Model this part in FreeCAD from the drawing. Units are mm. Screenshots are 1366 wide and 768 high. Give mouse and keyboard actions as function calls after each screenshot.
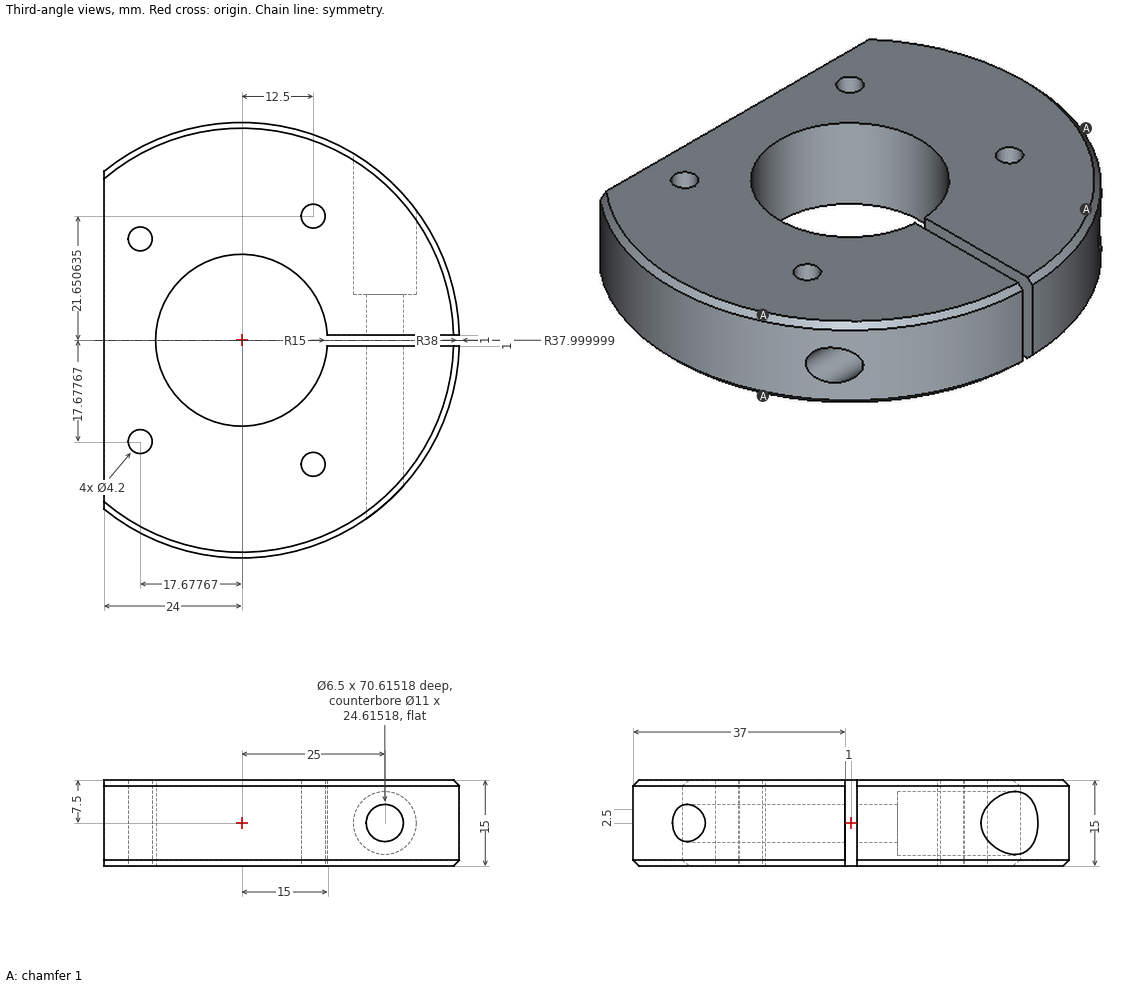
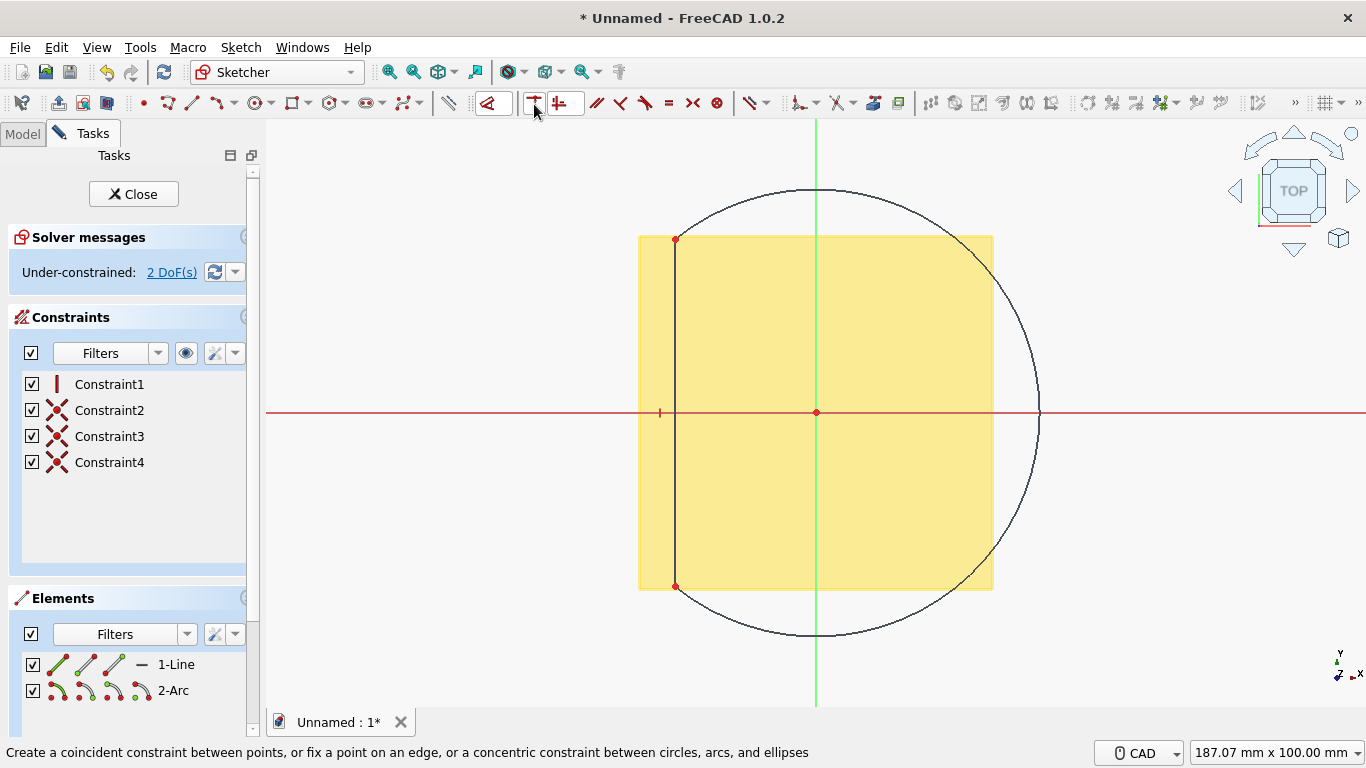
click(488, 104)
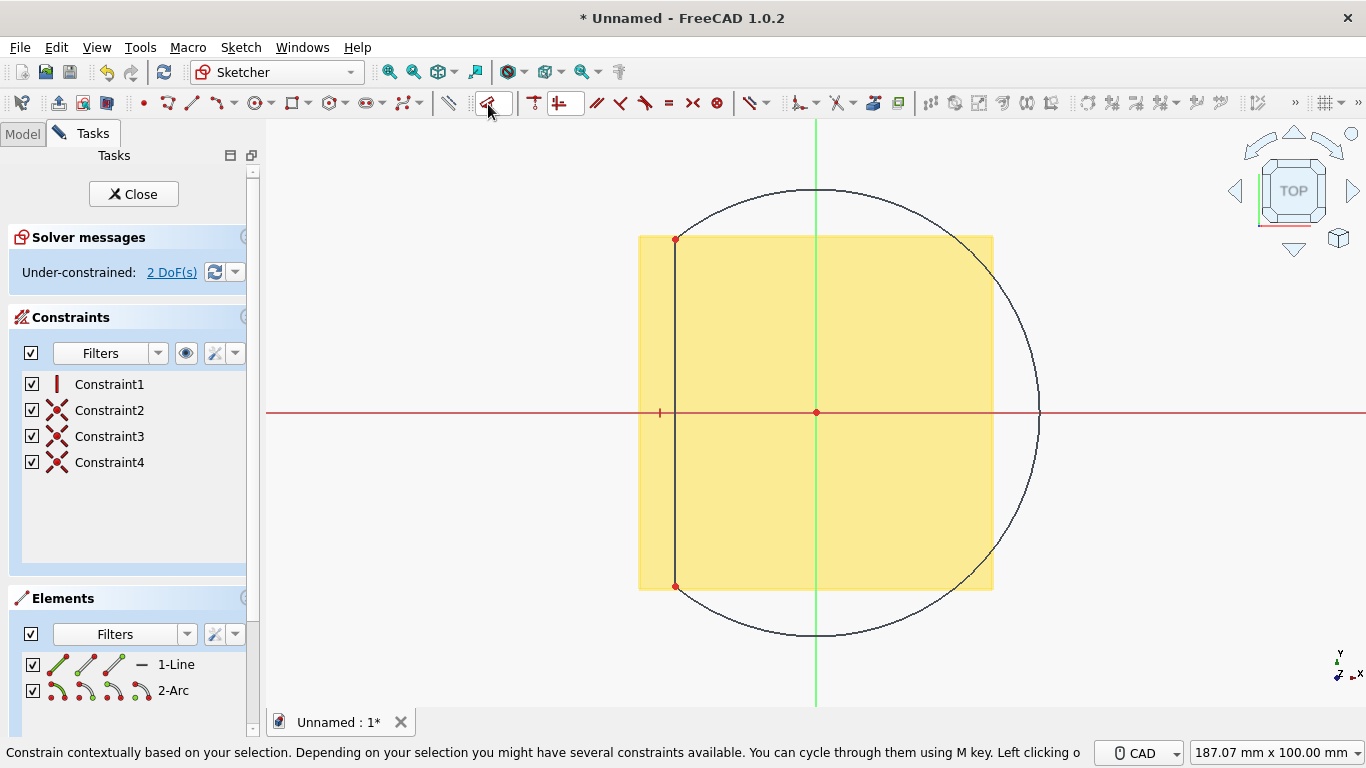
click(955, 588)
click(975, 613)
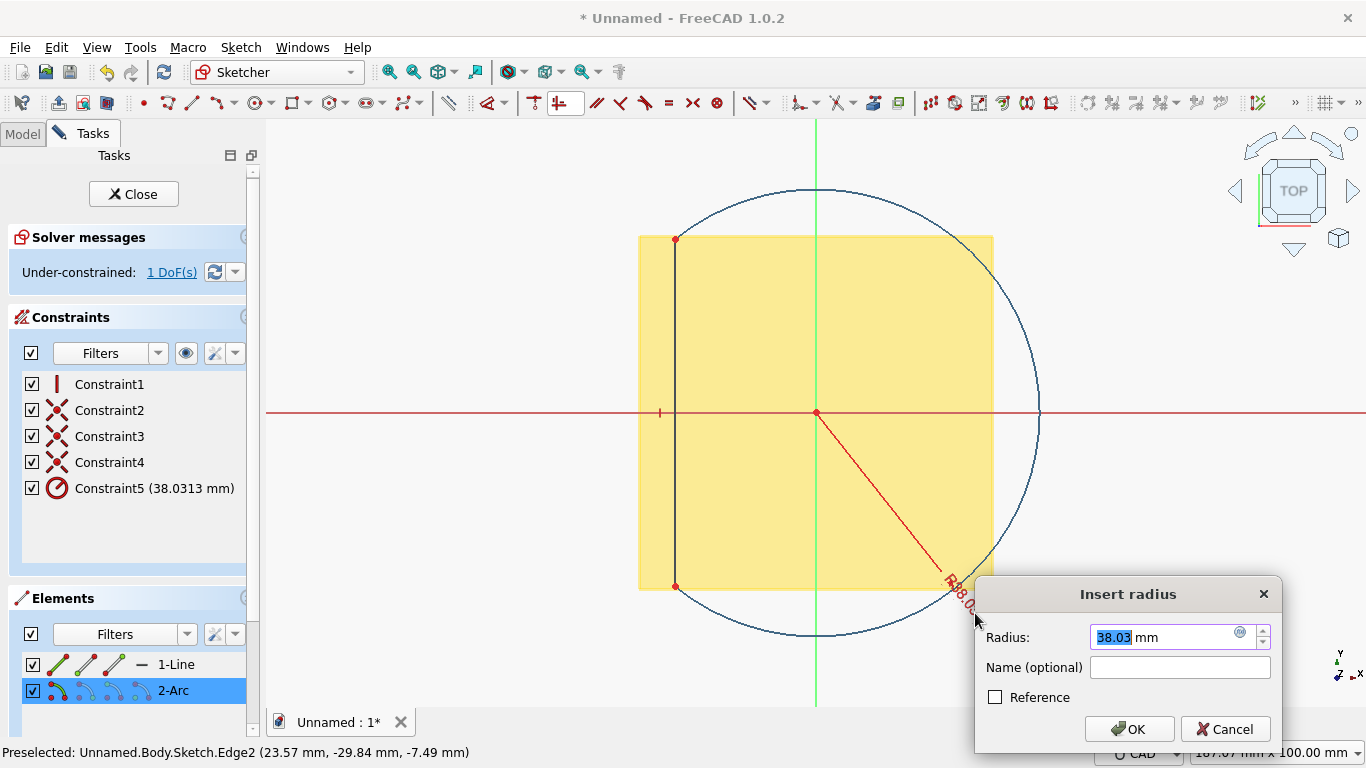
text(38)
key(Return)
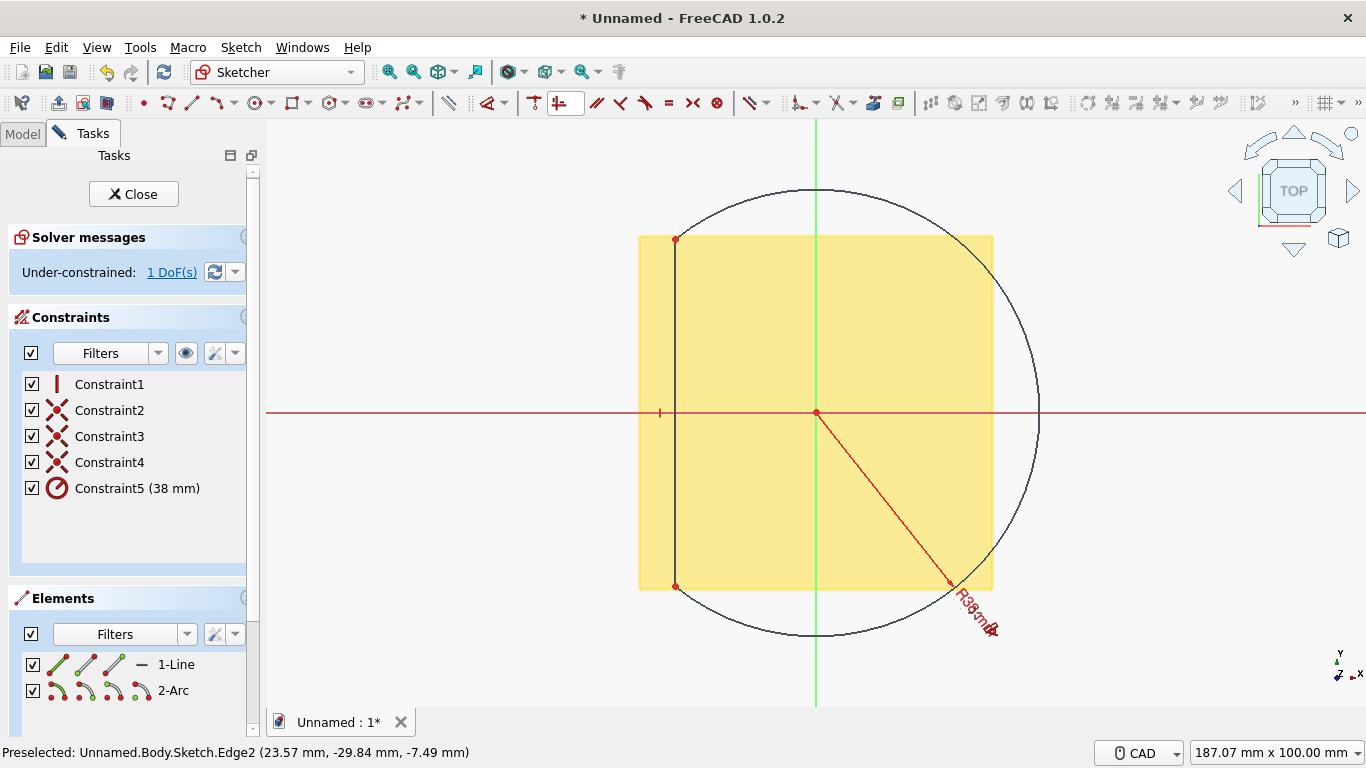
click(675, 587)
click(696, 621)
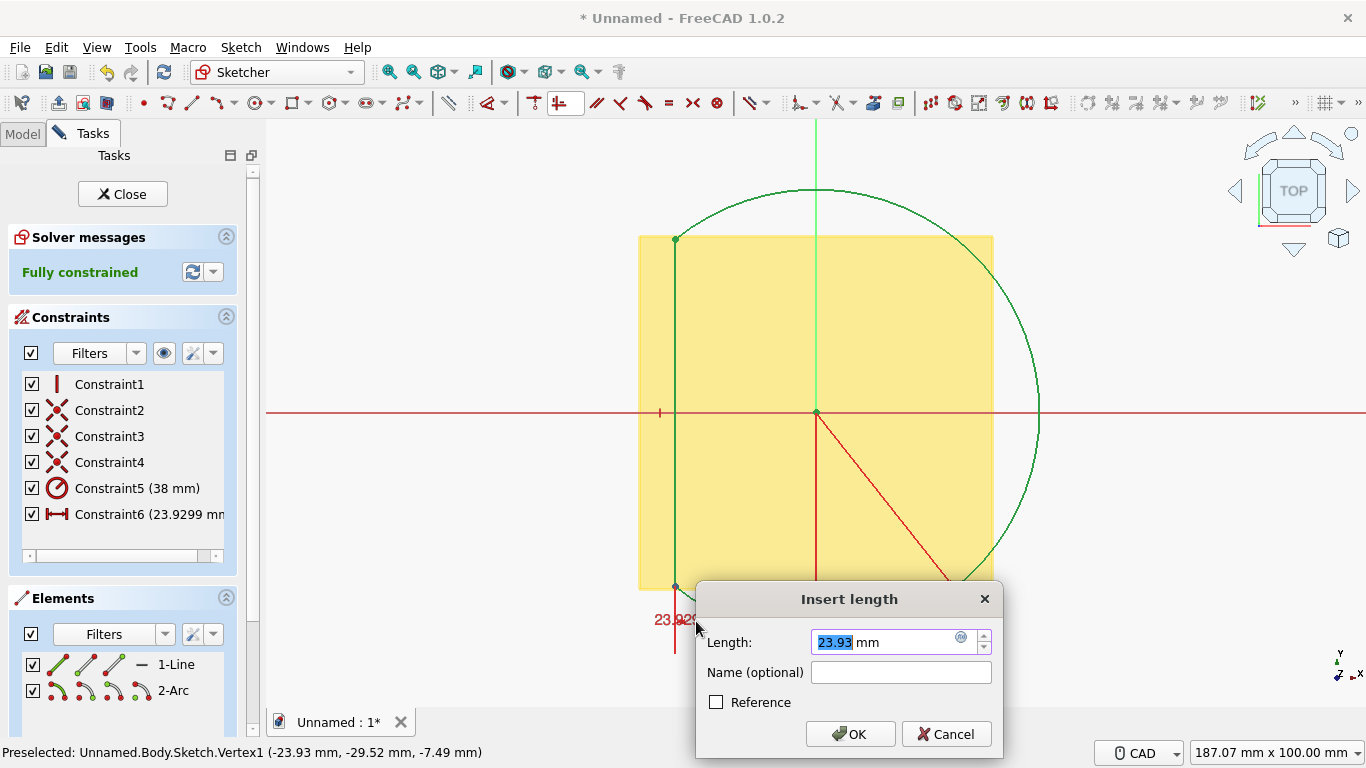
text(24)
key(Return)
key(Escape)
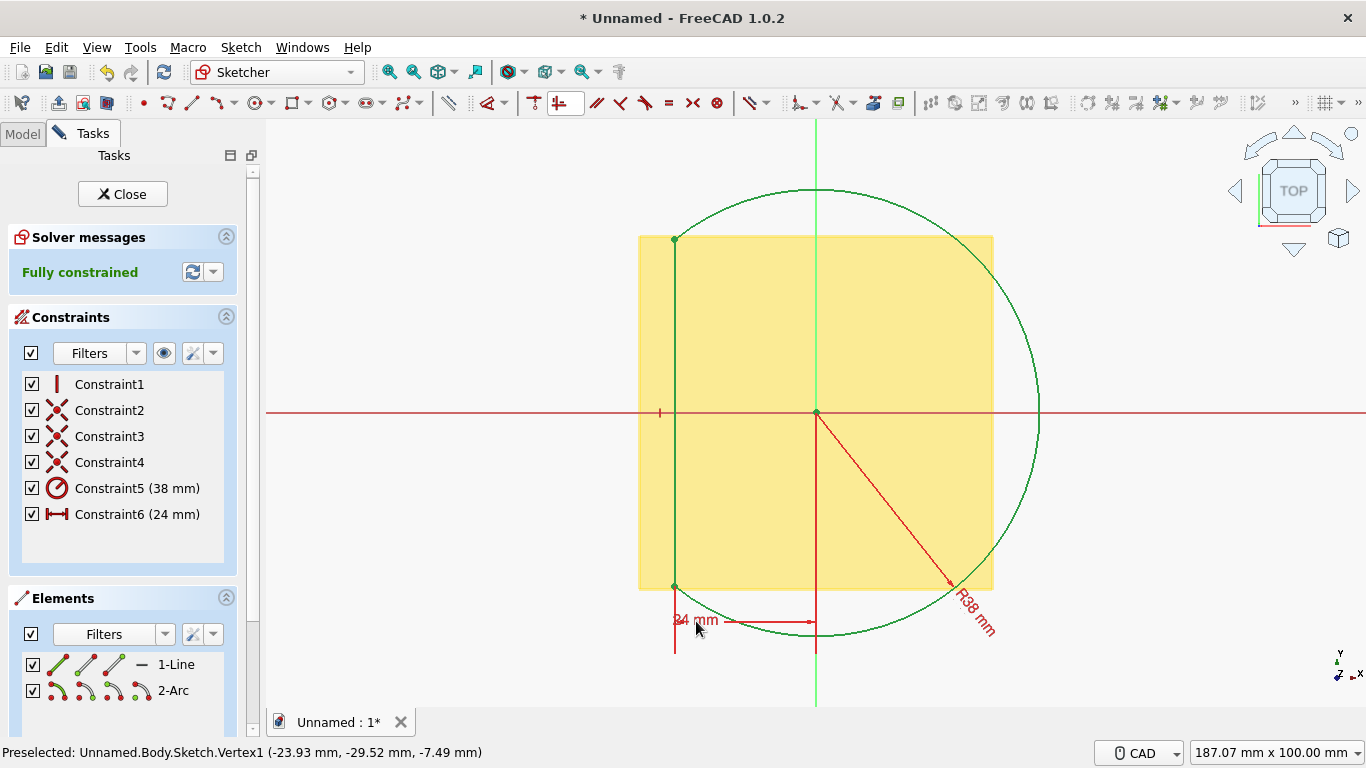
click(123, 194)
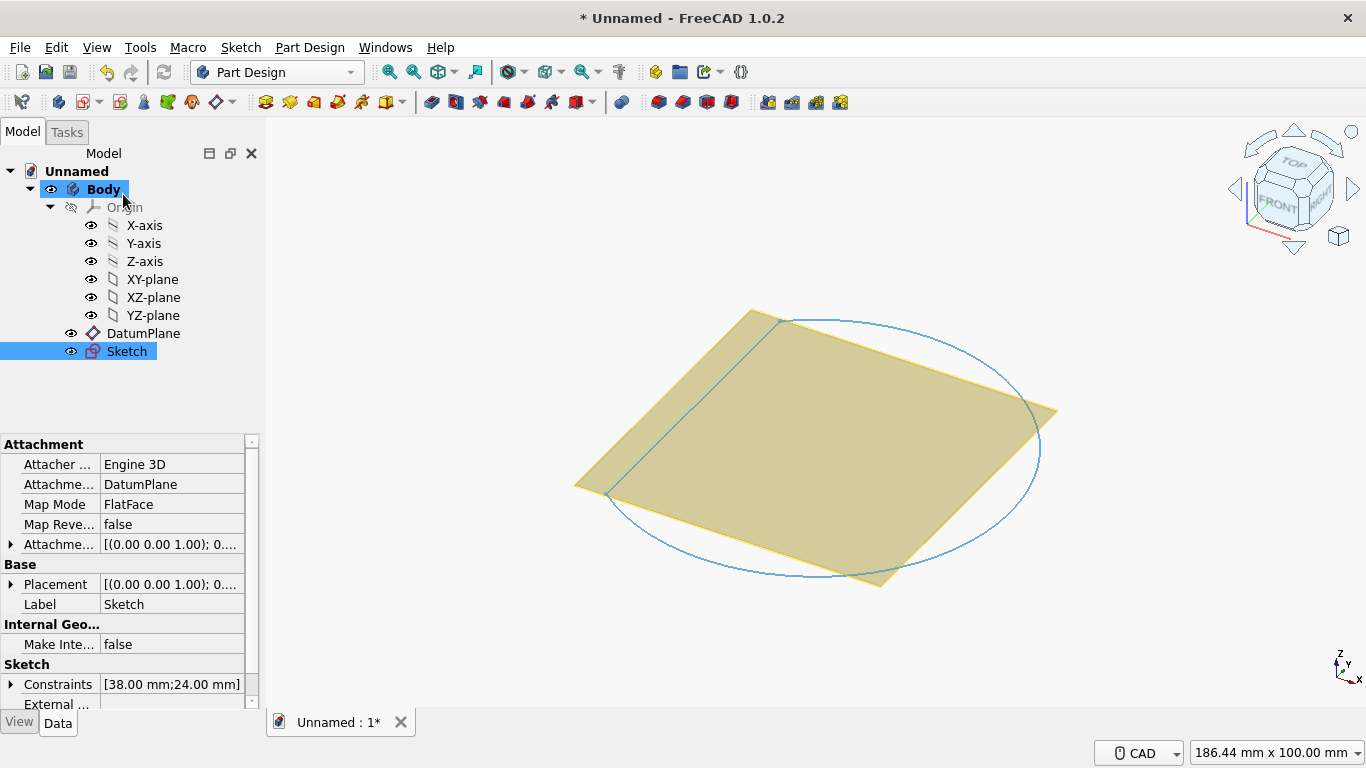
click(266, 102)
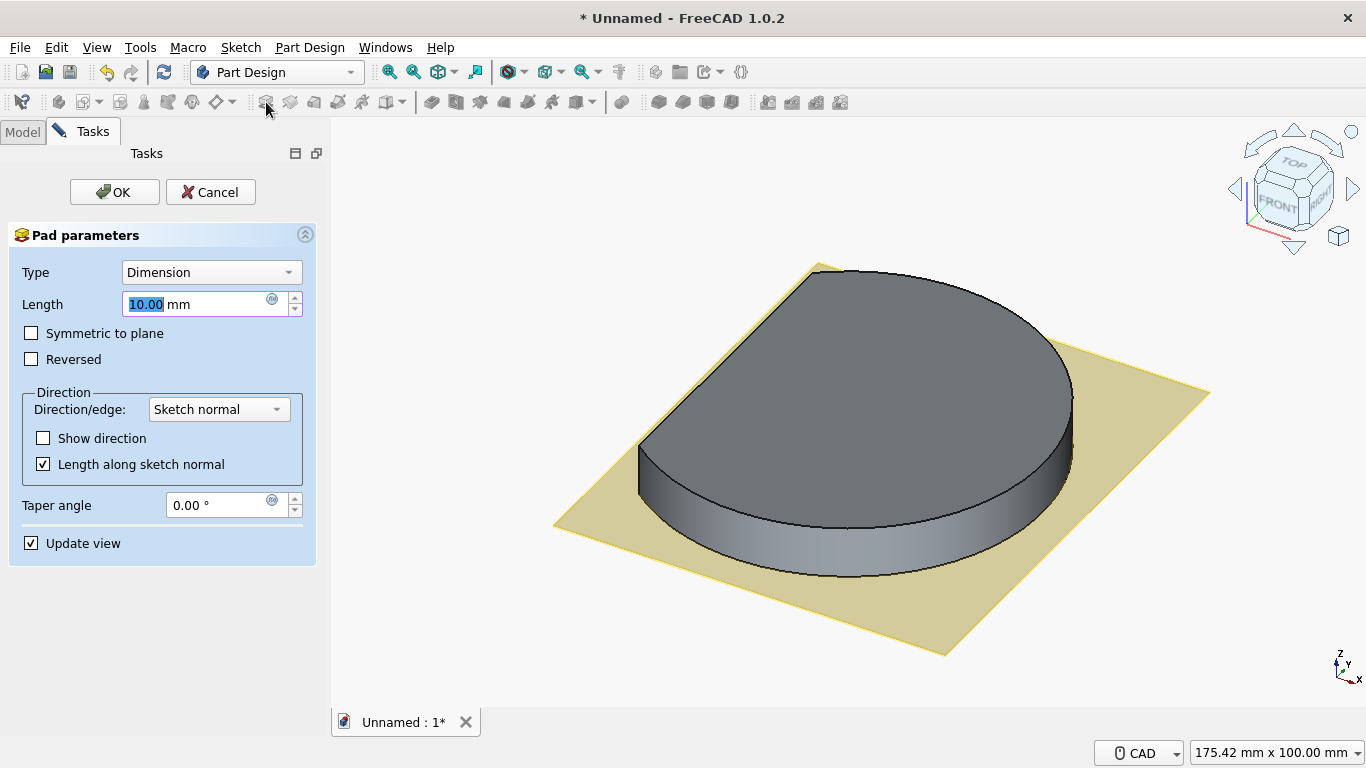
text(15)
key(Tab)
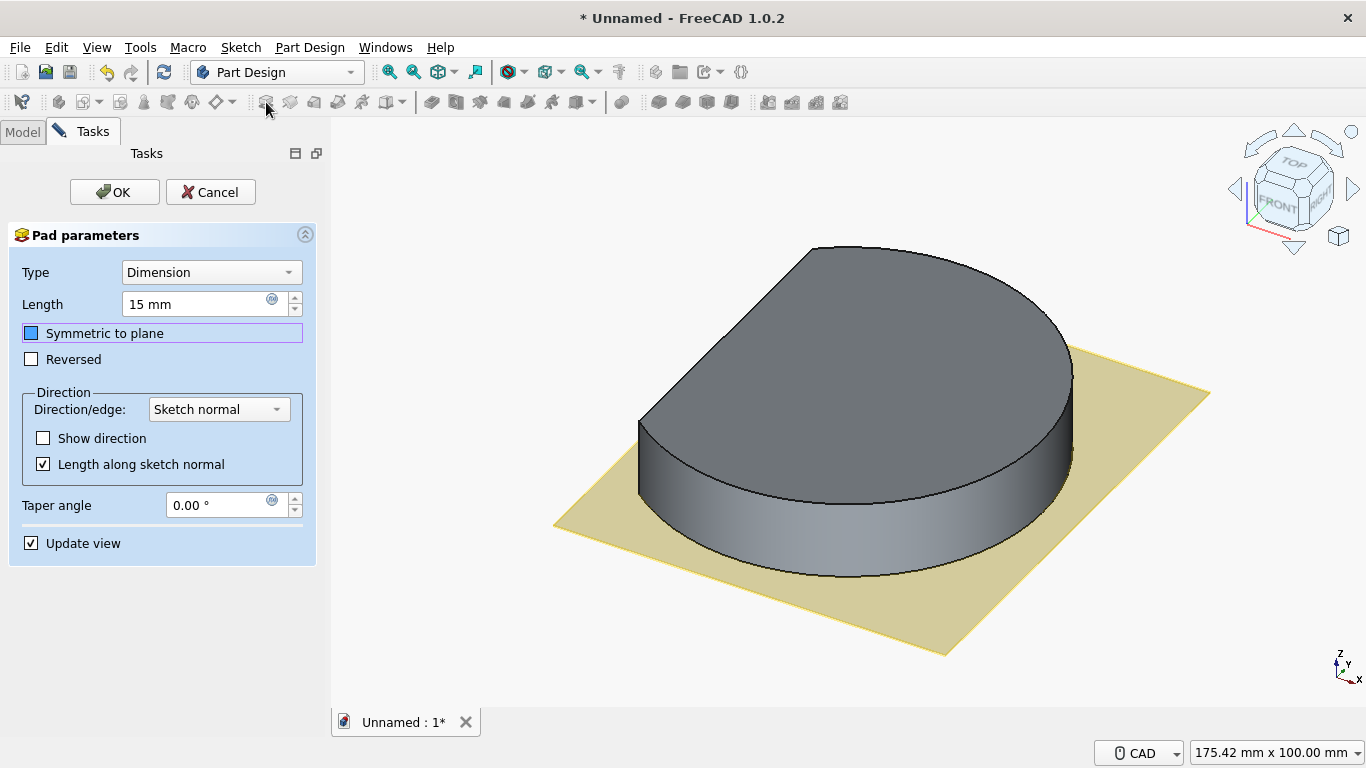
click(115, 192)